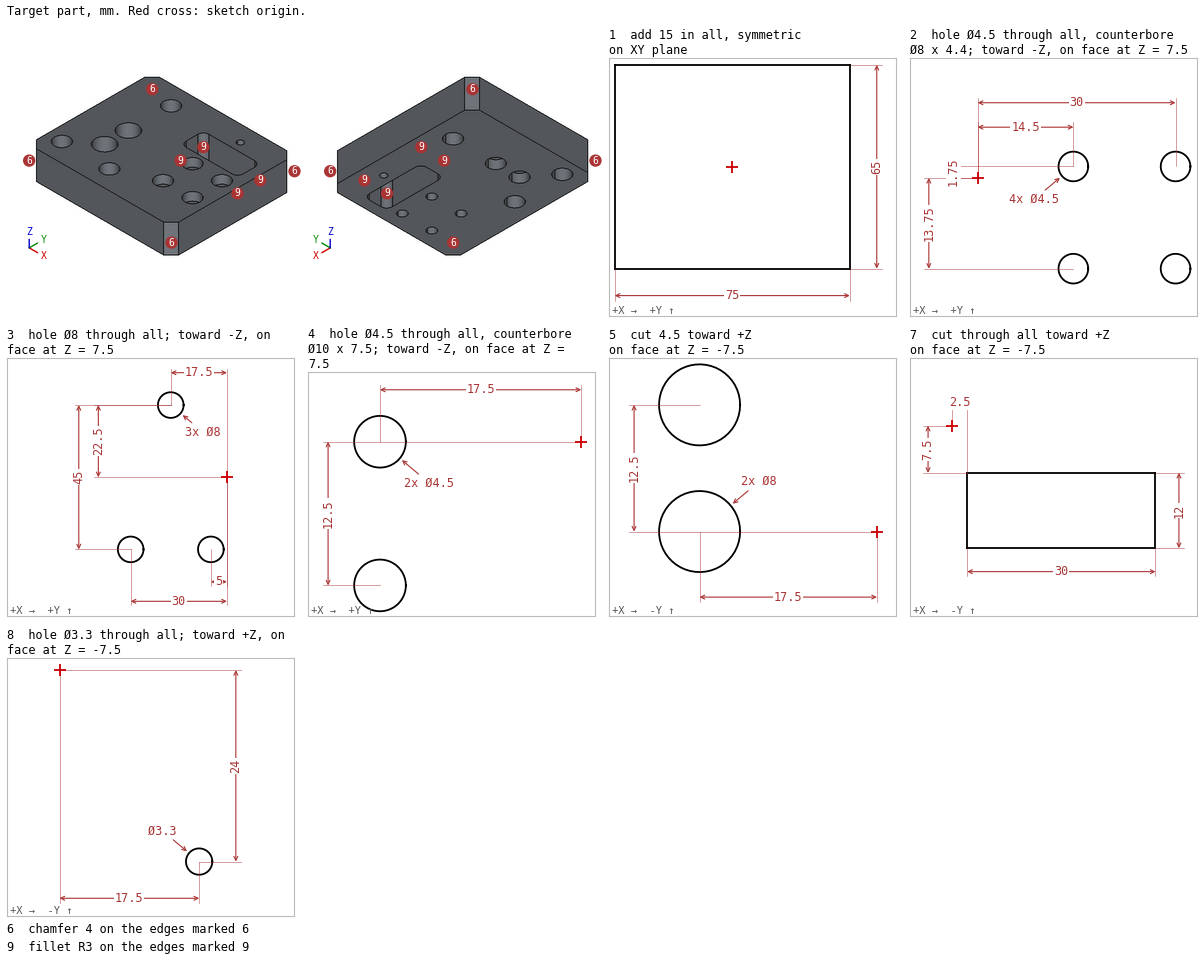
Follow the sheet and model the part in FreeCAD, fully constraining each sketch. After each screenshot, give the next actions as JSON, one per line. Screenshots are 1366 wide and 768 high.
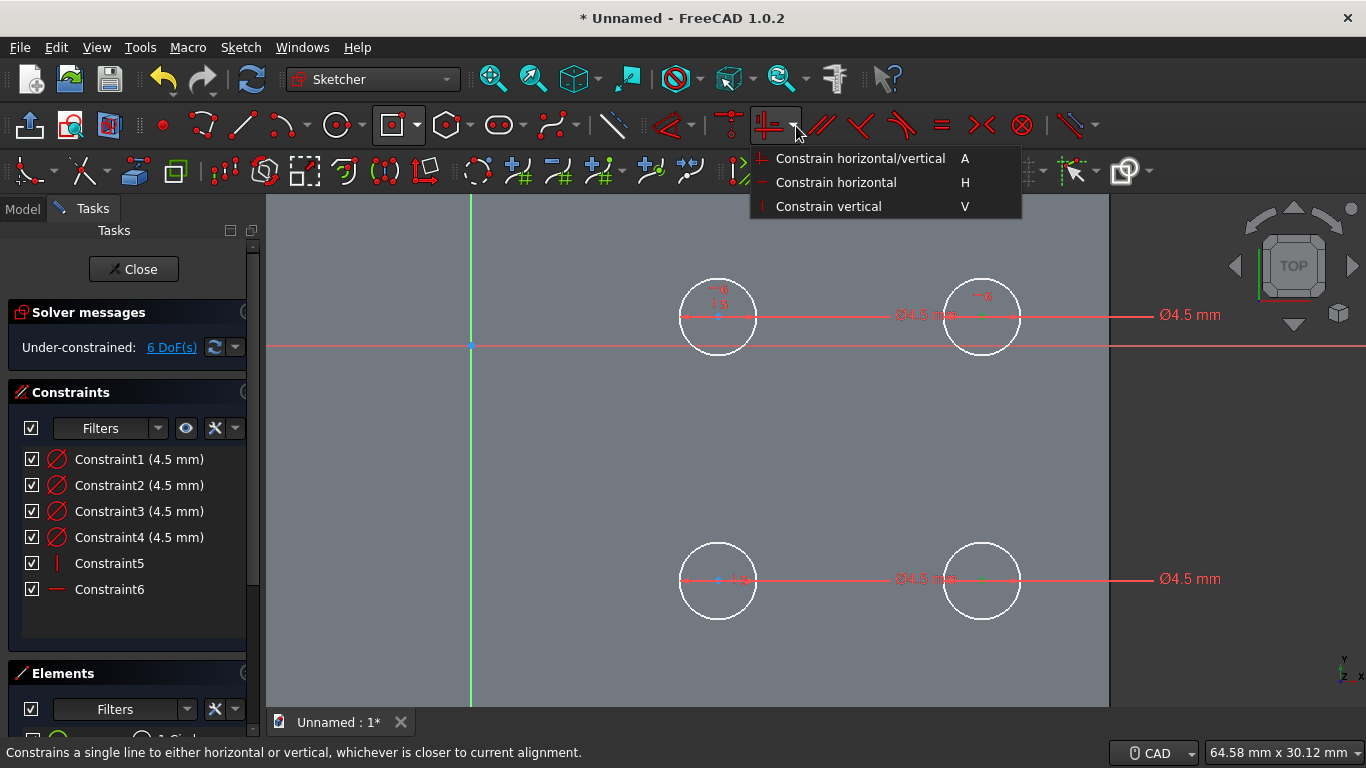
{"action": "left_click", "coordinate": [886, 206]}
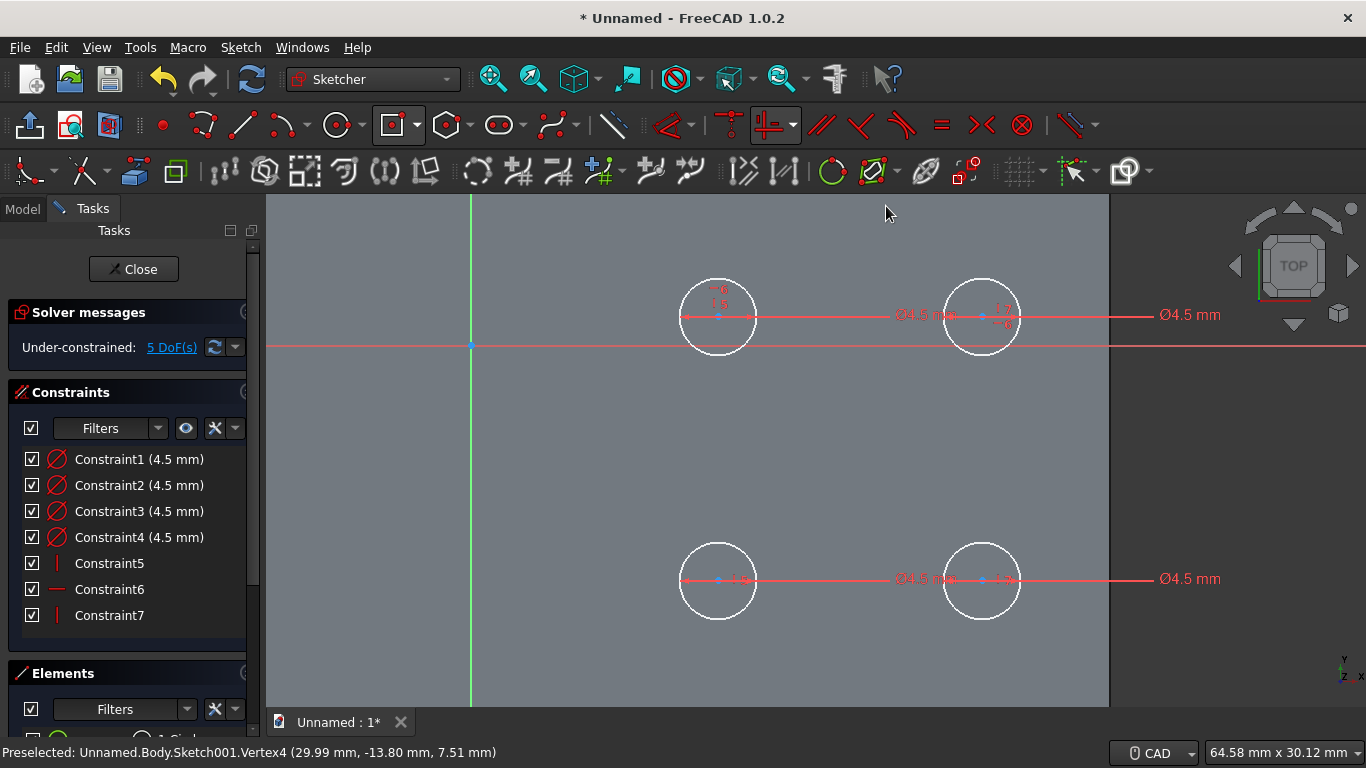
{"action": "left_click", "coordinate": [718, 581]}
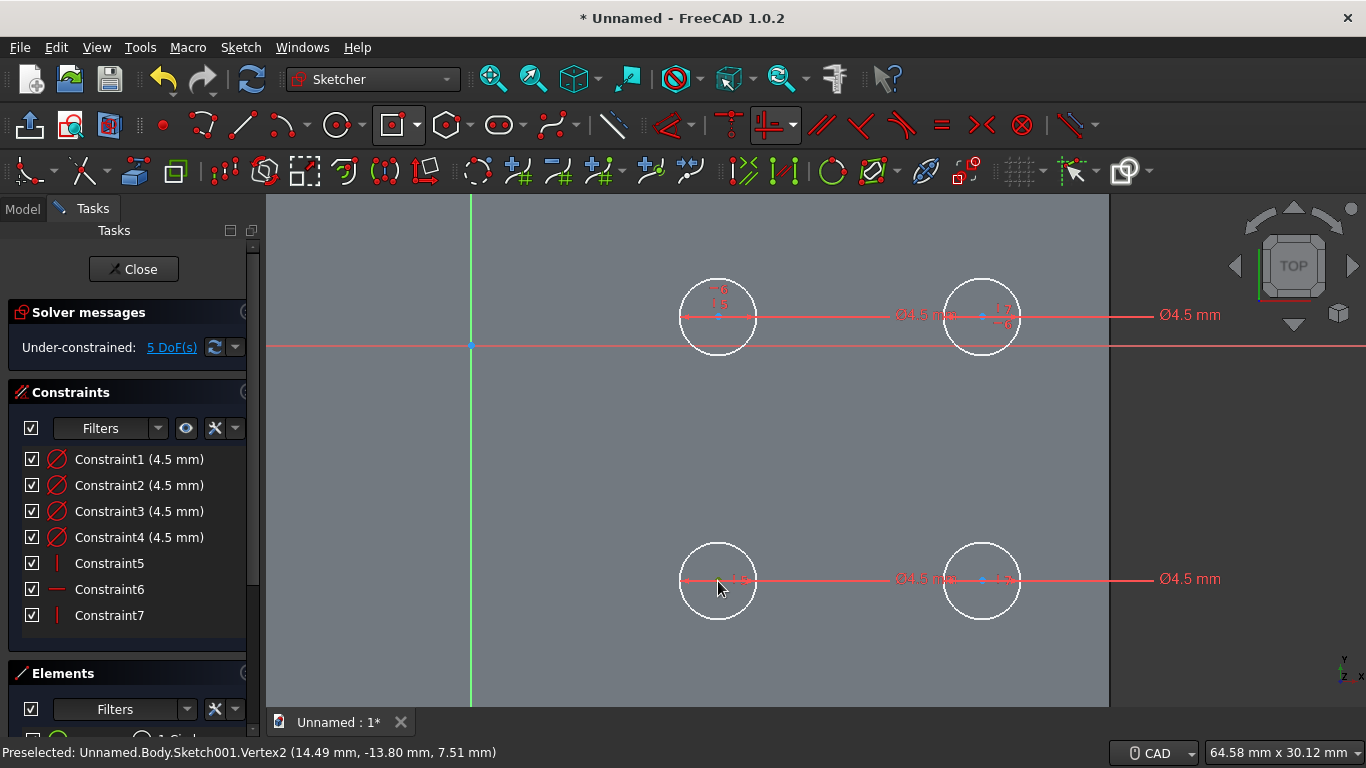
{"action": "left_click", "coordinate": [982, 581]}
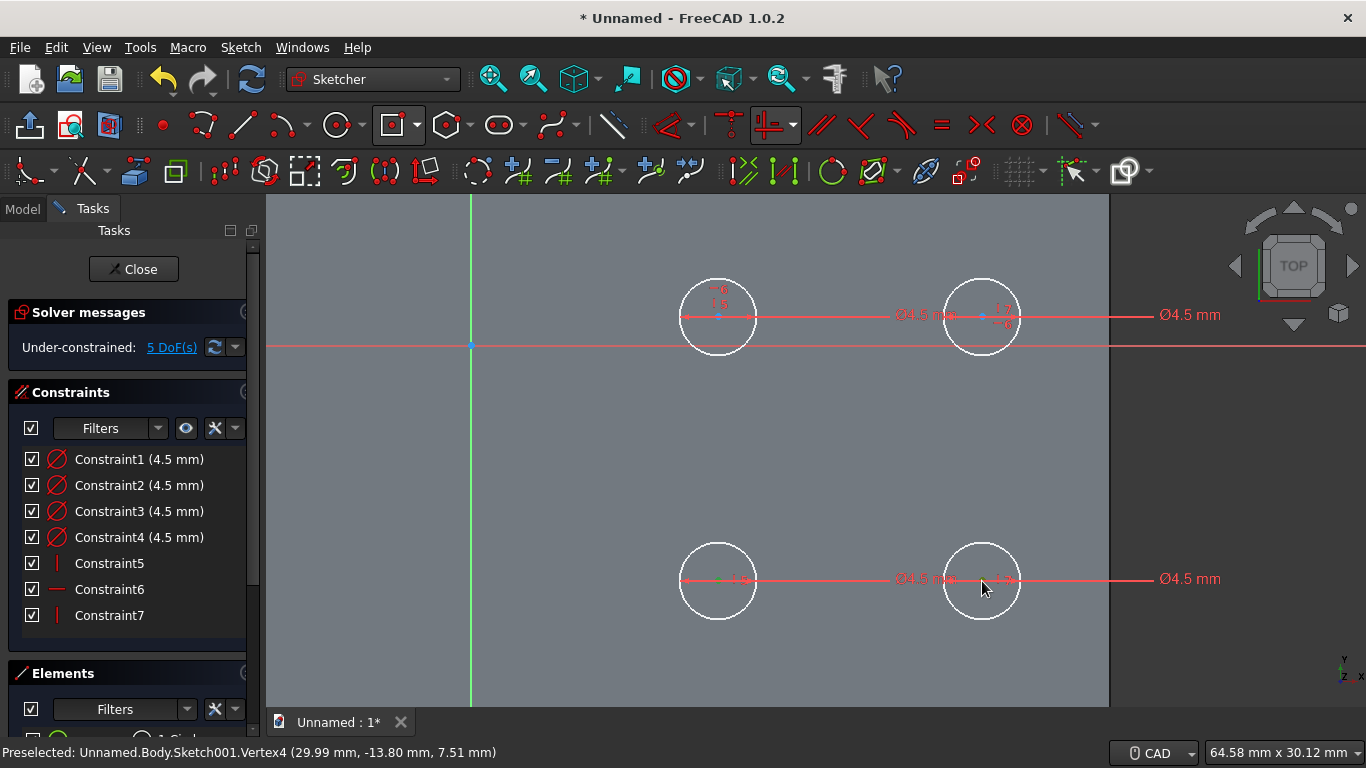
{"action": "key", "text": "h"}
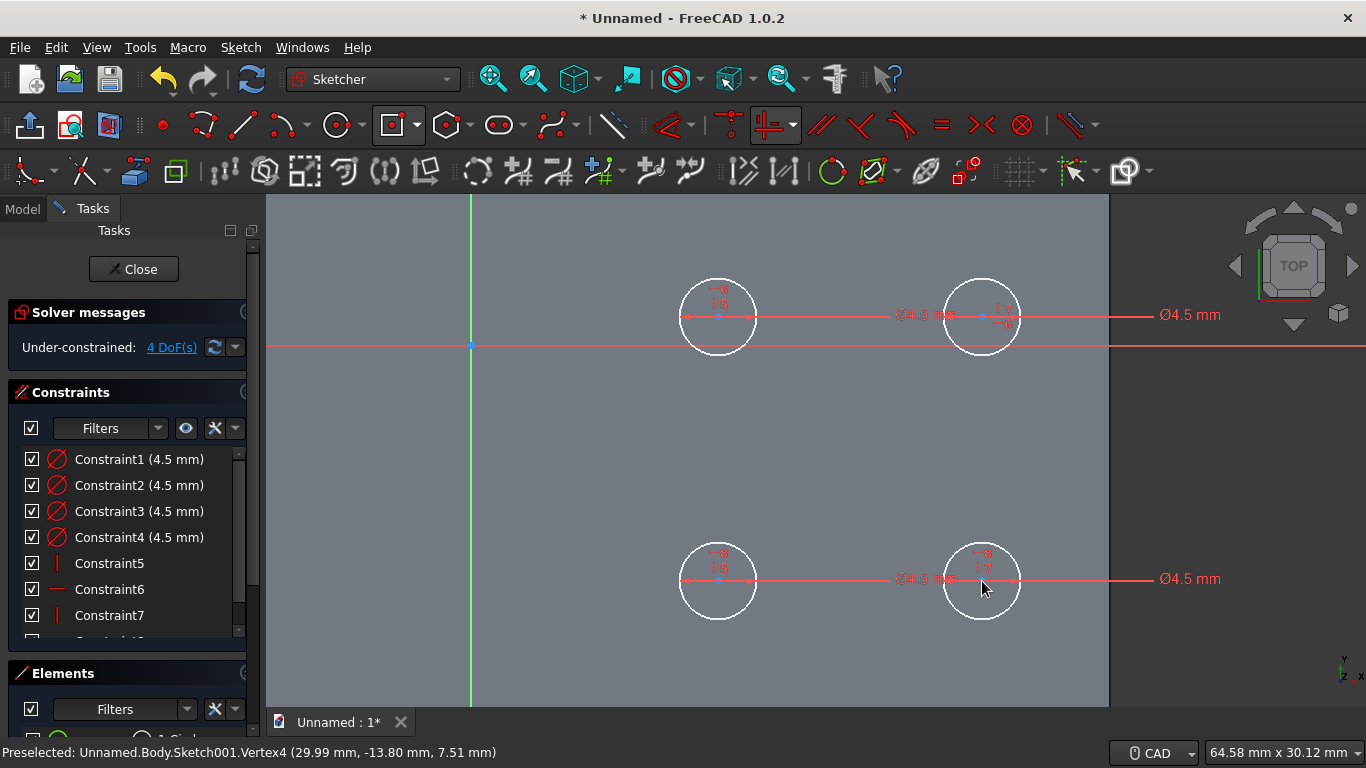
{"action": "left_click", "coordinate": [982, 317]}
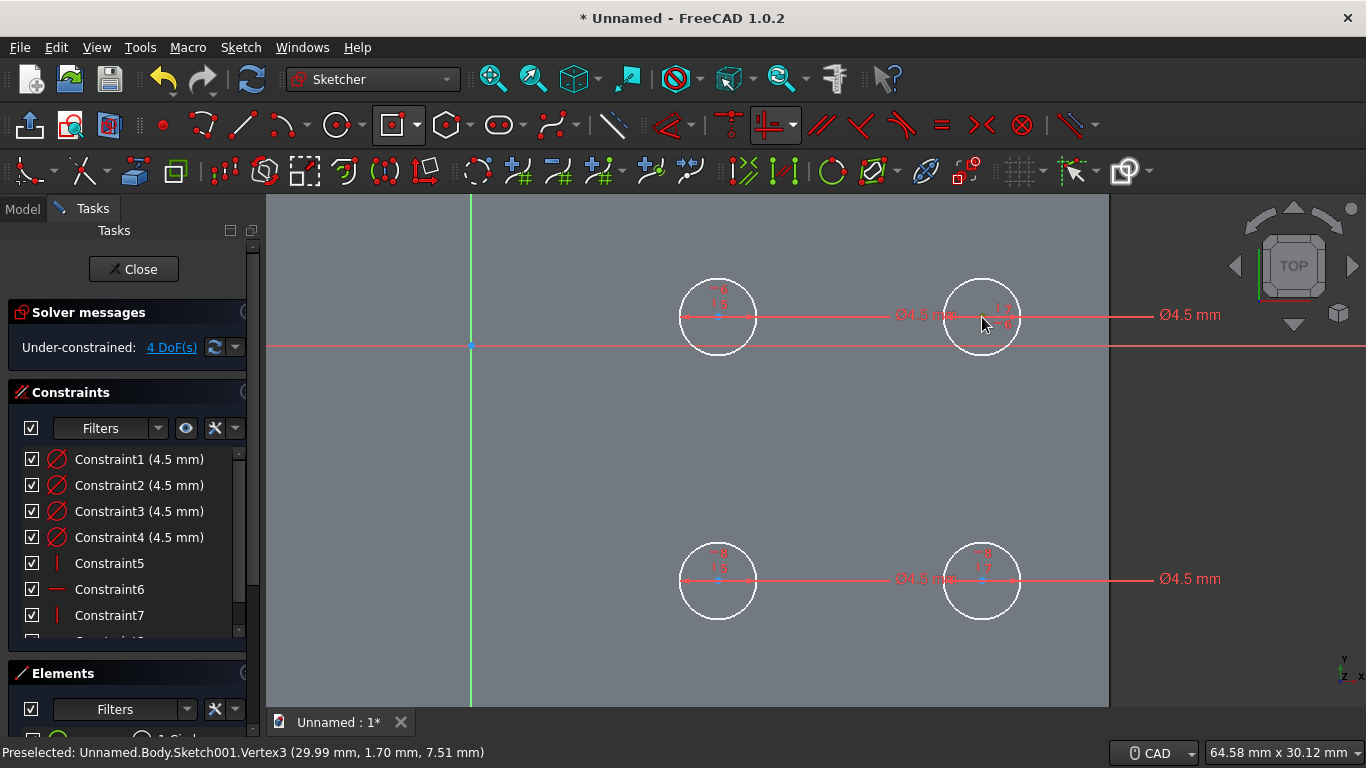
{"action": "key", "text": "l"}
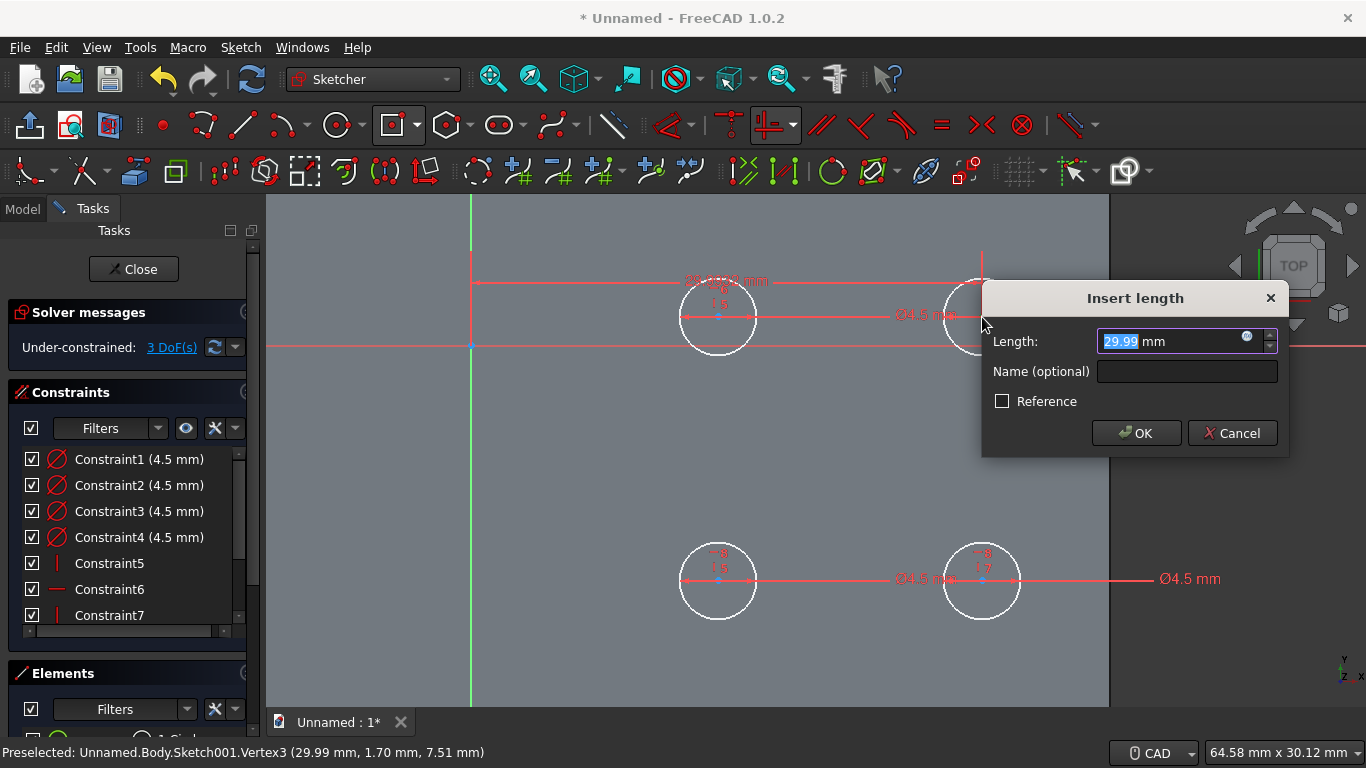
{"action": "type", "text": "30"}
{"action": "key", "text": "Return"}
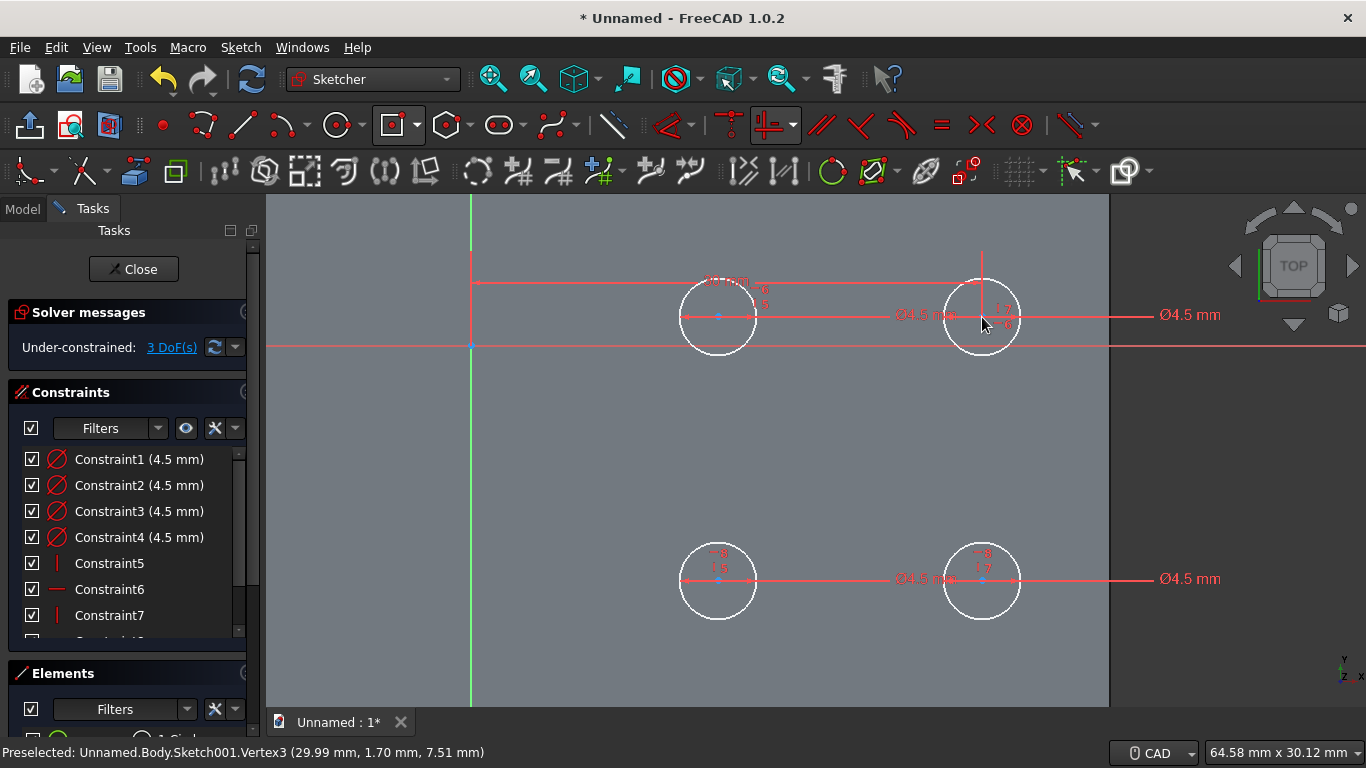
{"action": "left_click", "coordinate": [718, 317]}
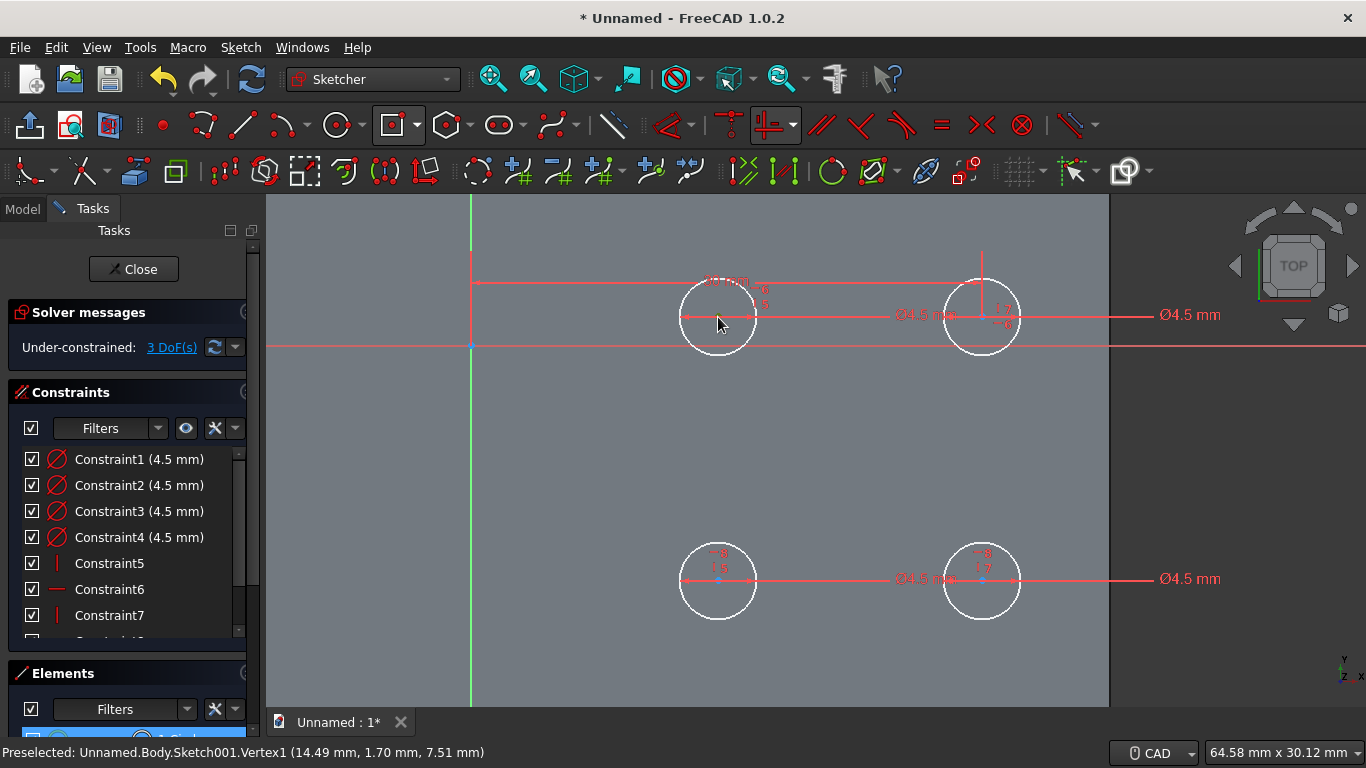
{"action": "key", "text": "l"}